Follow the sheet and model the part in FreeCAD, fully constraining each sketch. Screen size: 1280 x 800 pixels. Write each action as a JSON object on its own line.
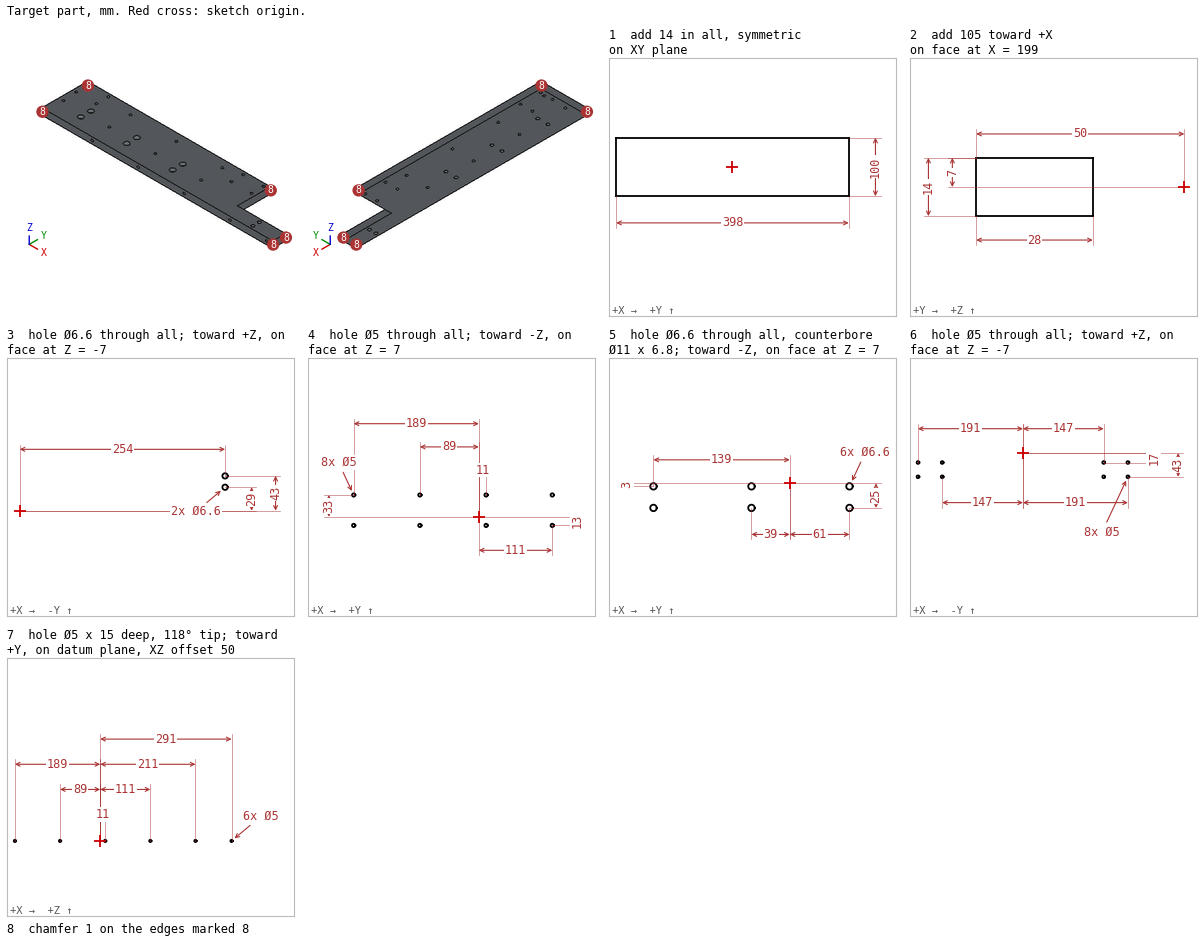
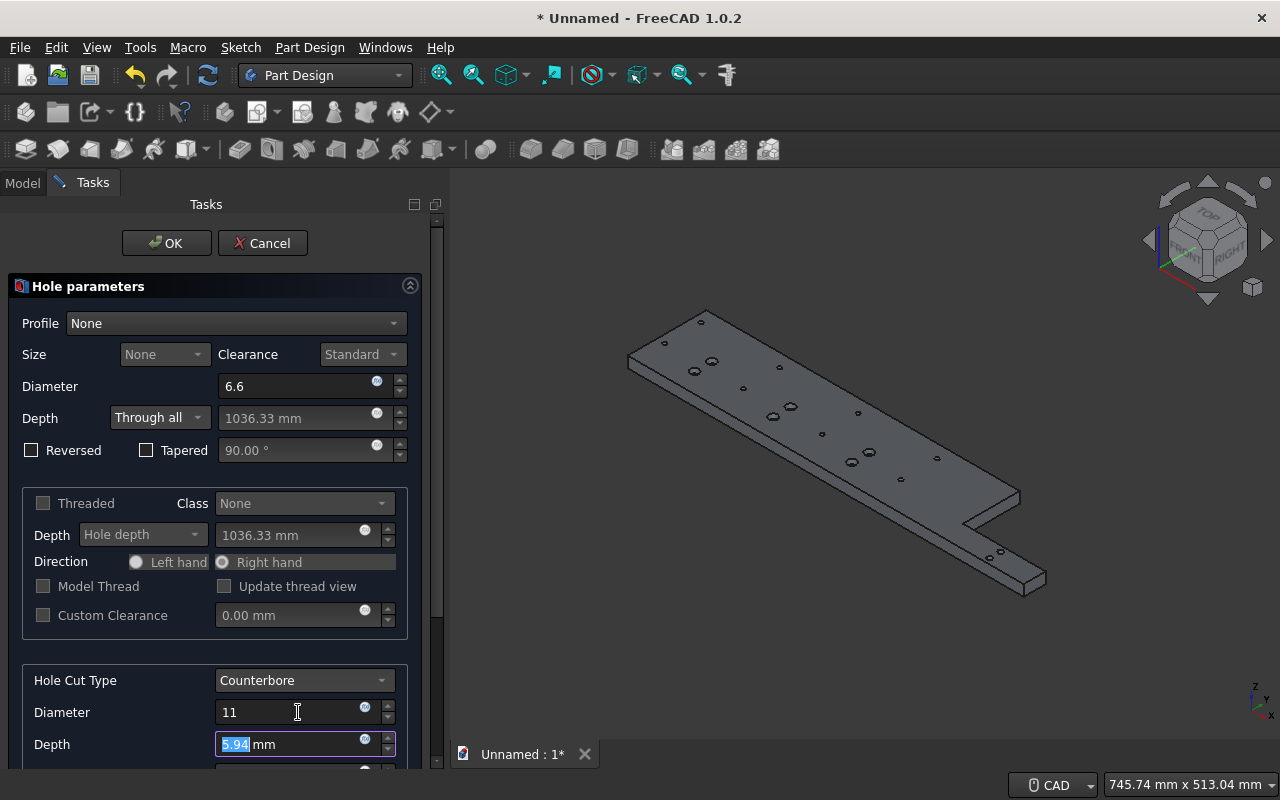
{"action": "type", "text": "6.8"}
{"action": "key", "text": "Tab"}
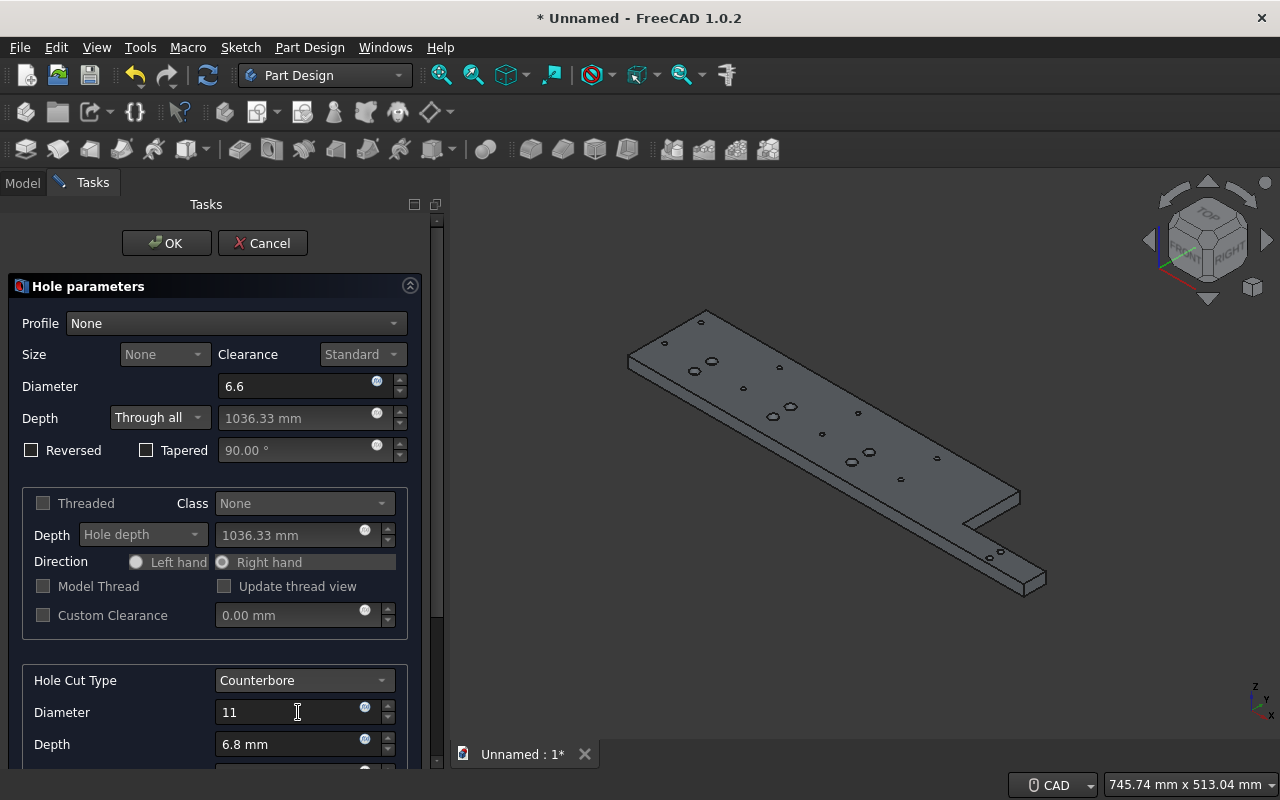
{"action": "left_click", "coordinate": [167, 243]}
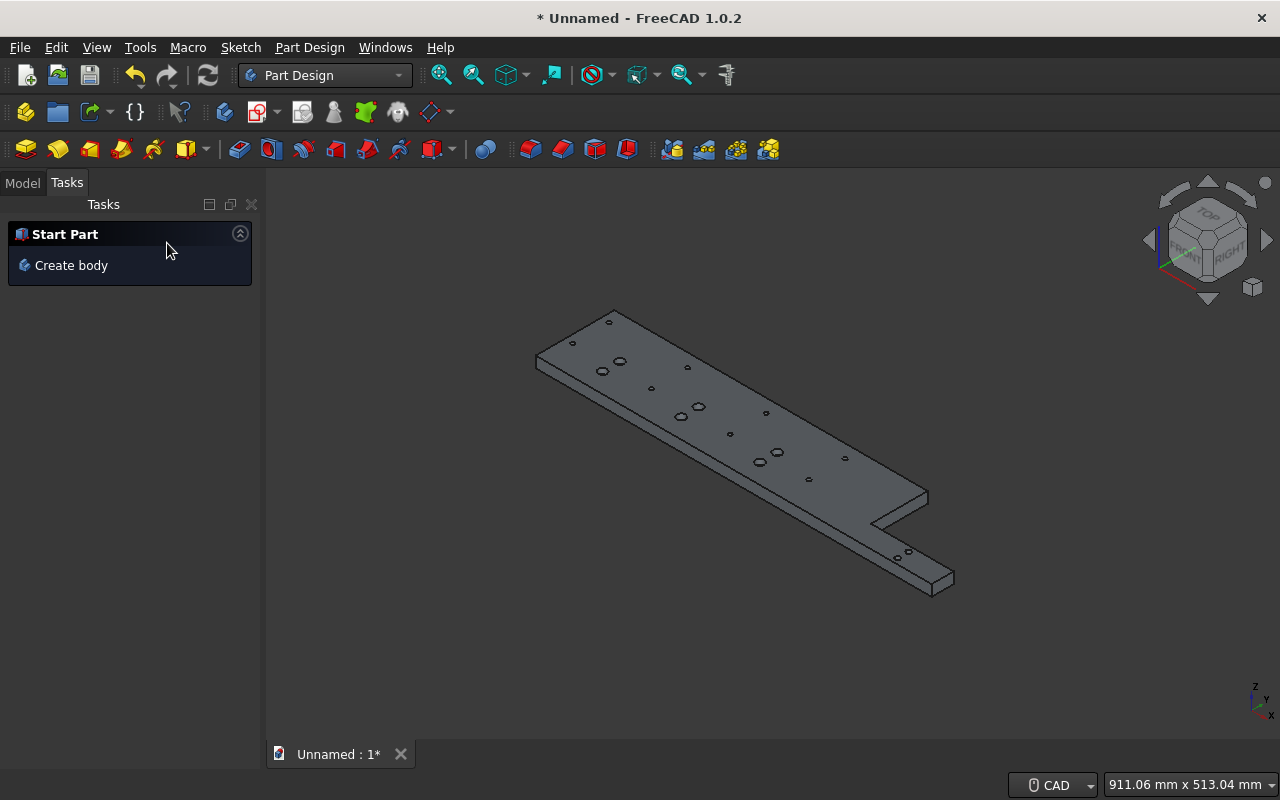
{"action": "key", "text": "5"}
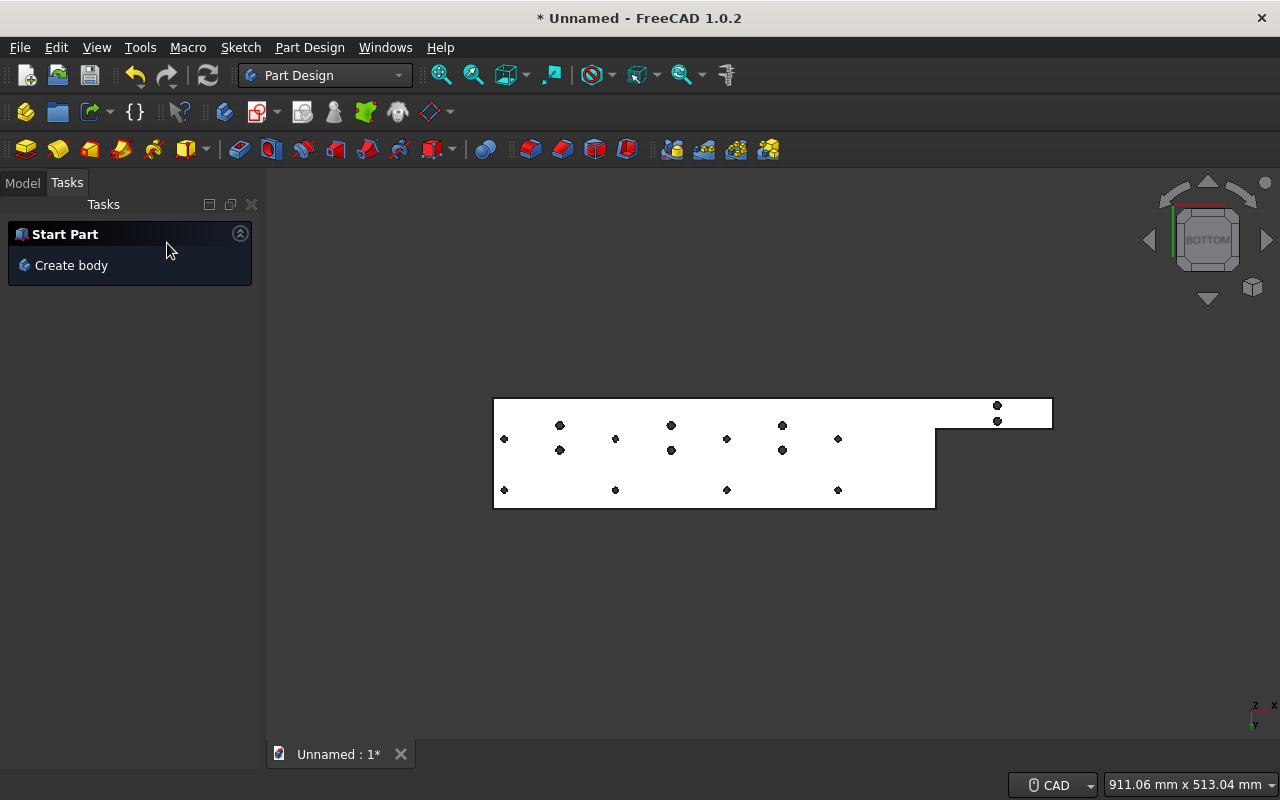
{"action": "left_click", "coordinate": [533, 468]}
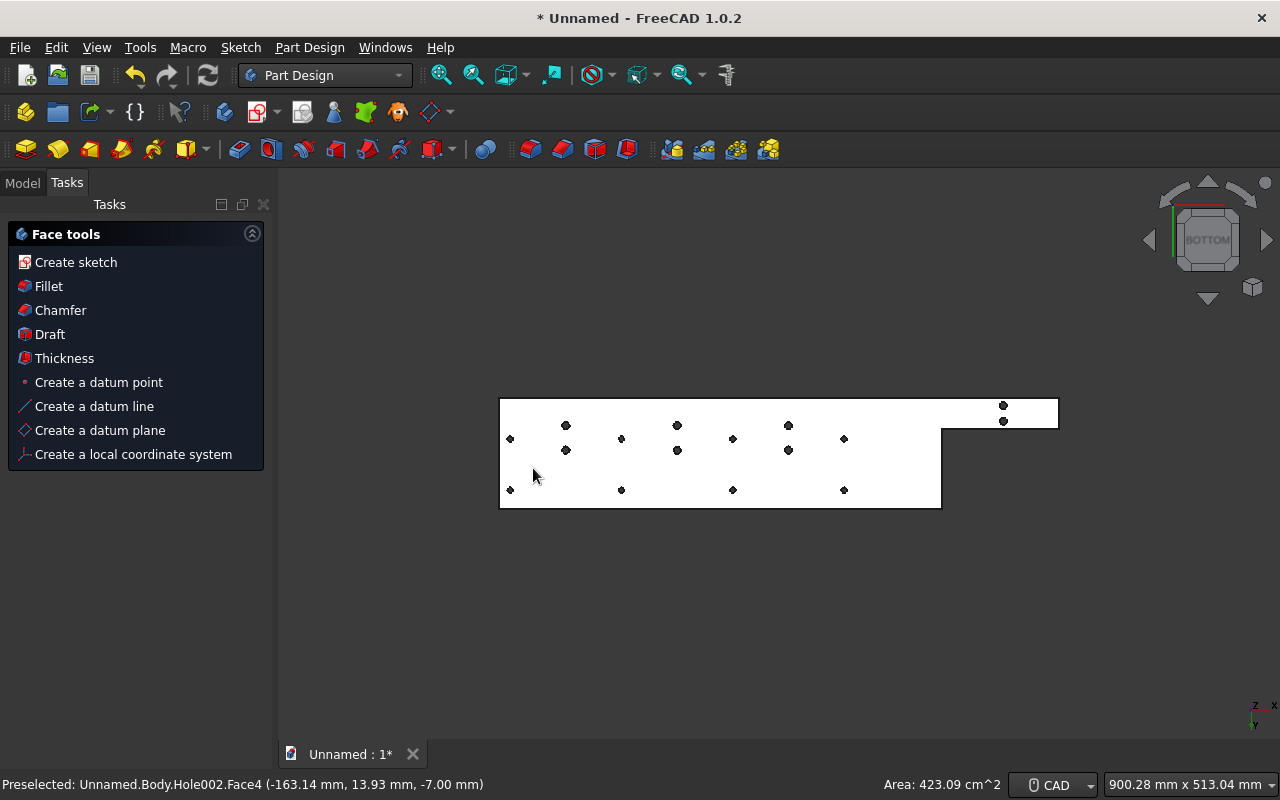
{"action": "left_click", "coordinate": [258, 112]}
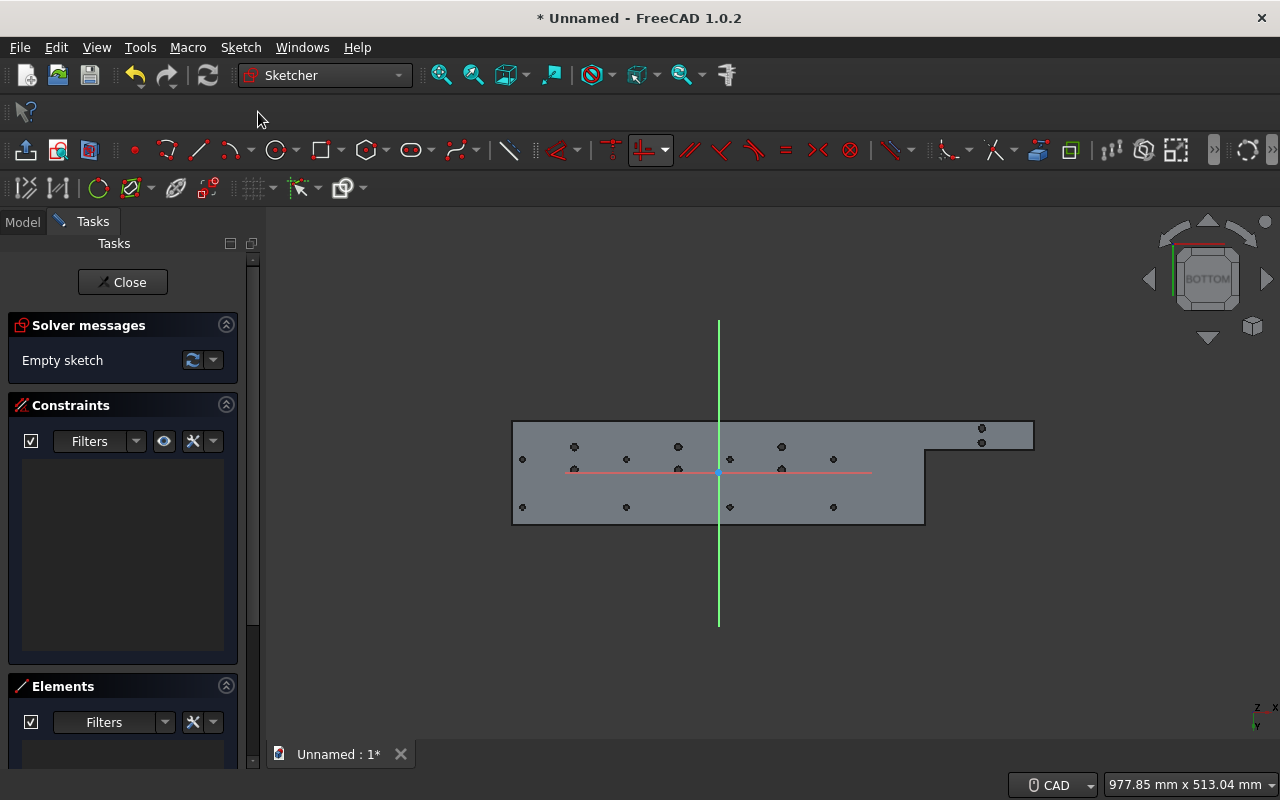
{"action": "scroll", "coordinate": [747, 545], "scroll_direction": "up", "scroll_amount": 2}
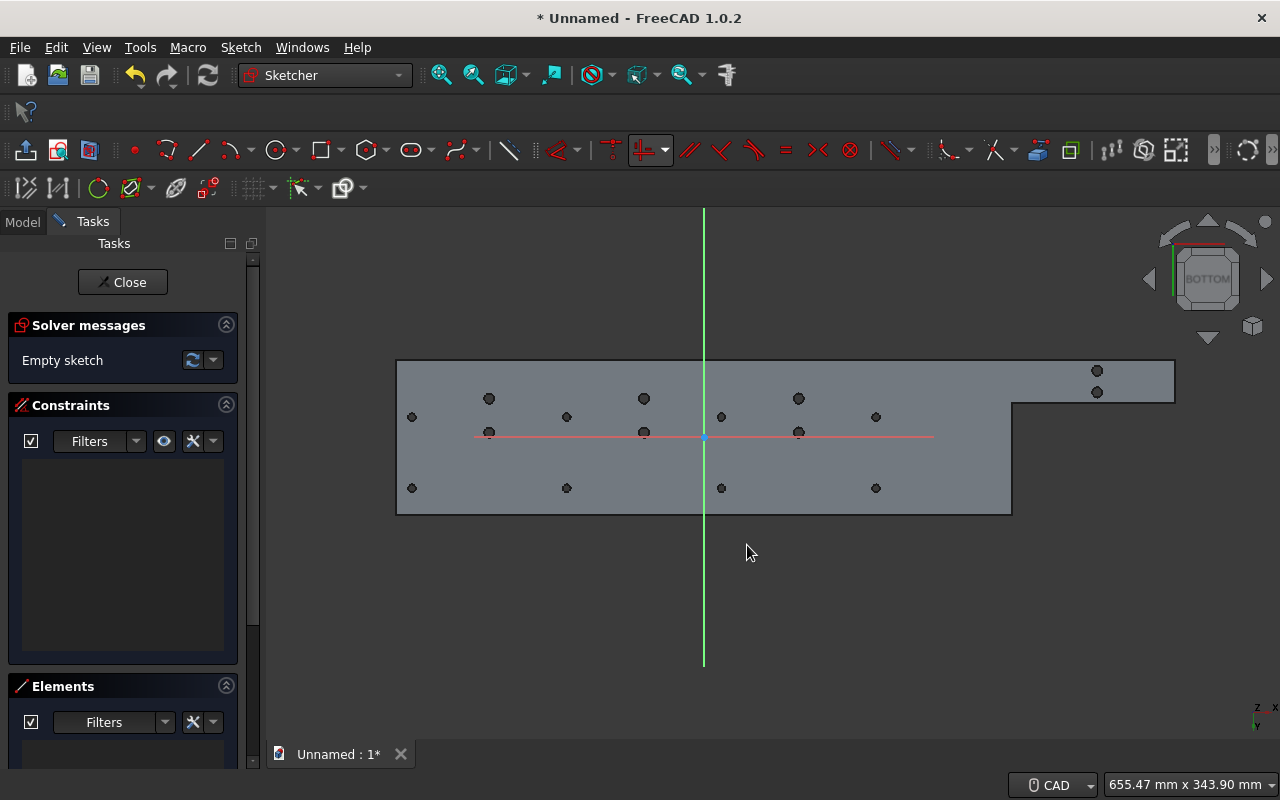
{"action": "key", "text": "g c"}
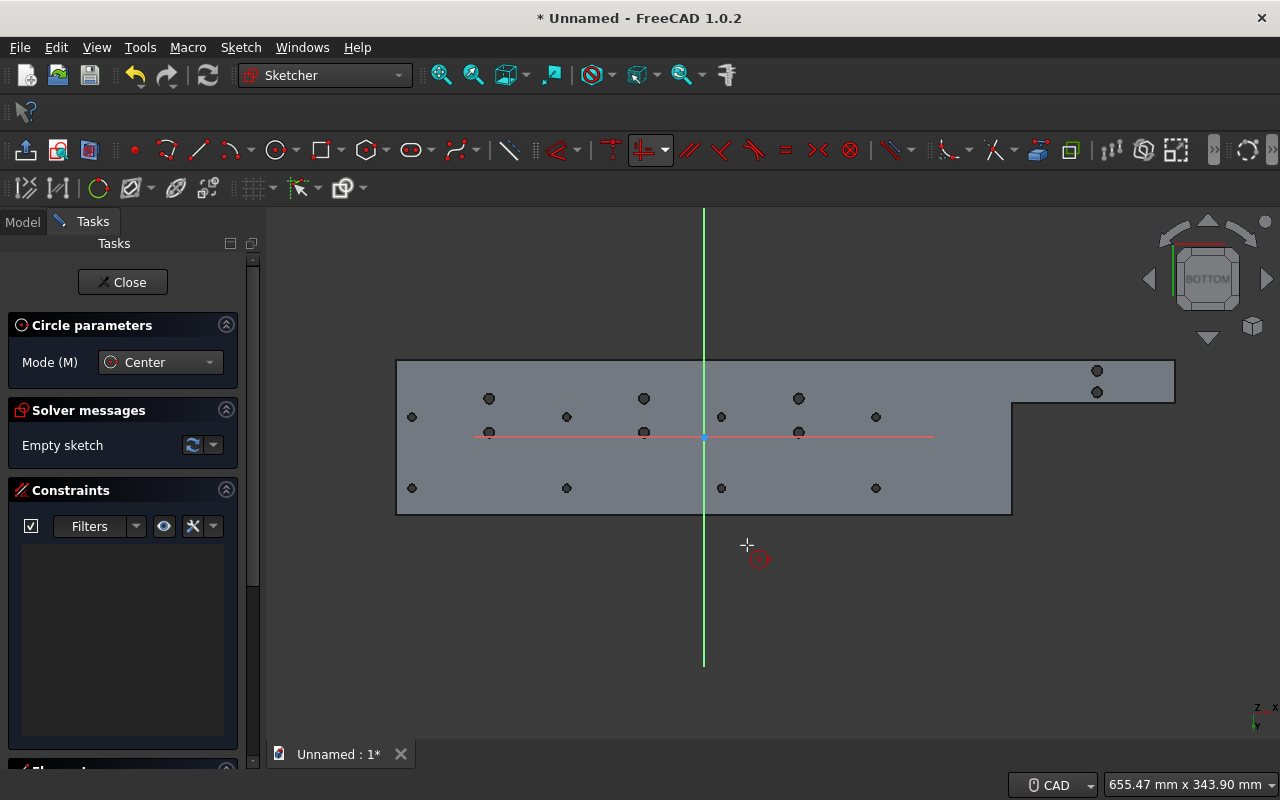
{"action": "scroll", "coordinate": [1000, 504], "scroll_direction": "up", "scroll_amount": 9}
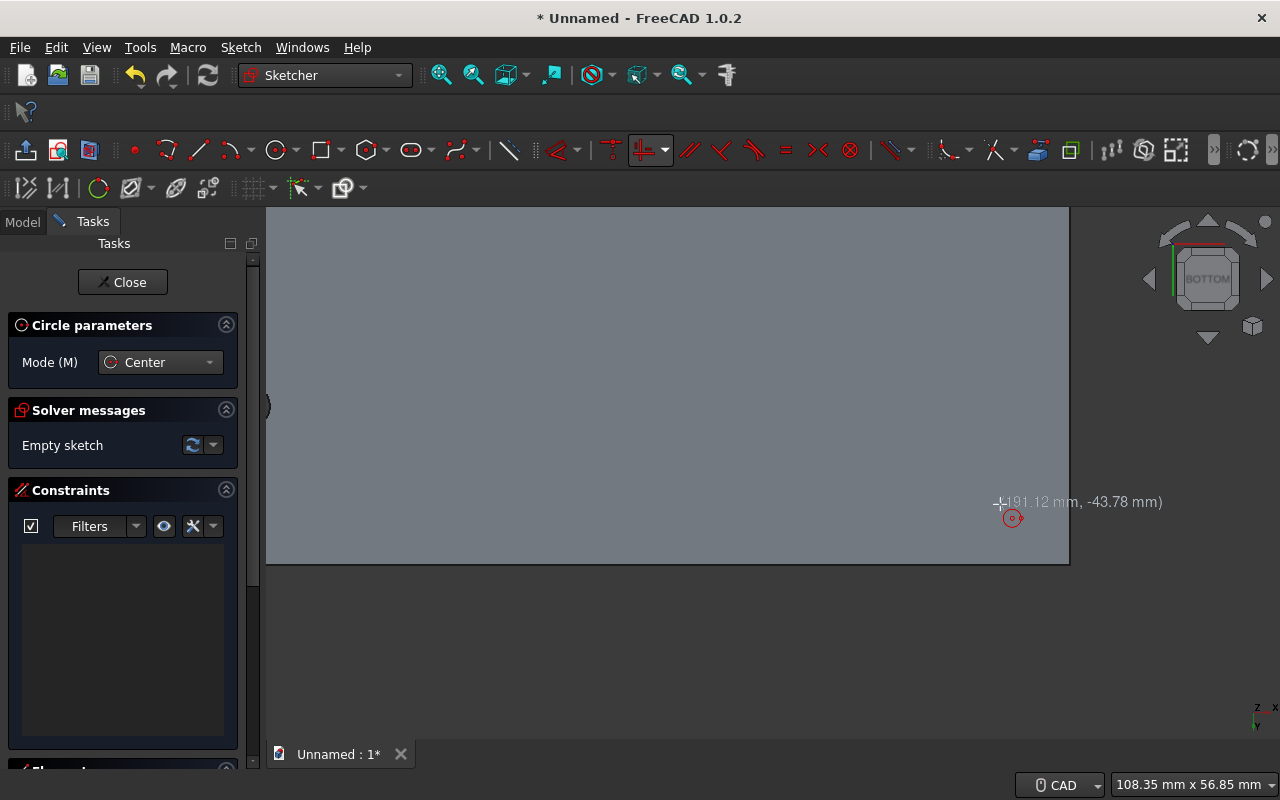
{"action": "scroll", "coordinate": [1001, 505], "scroll_direction": "down", "scroll_amount": 9}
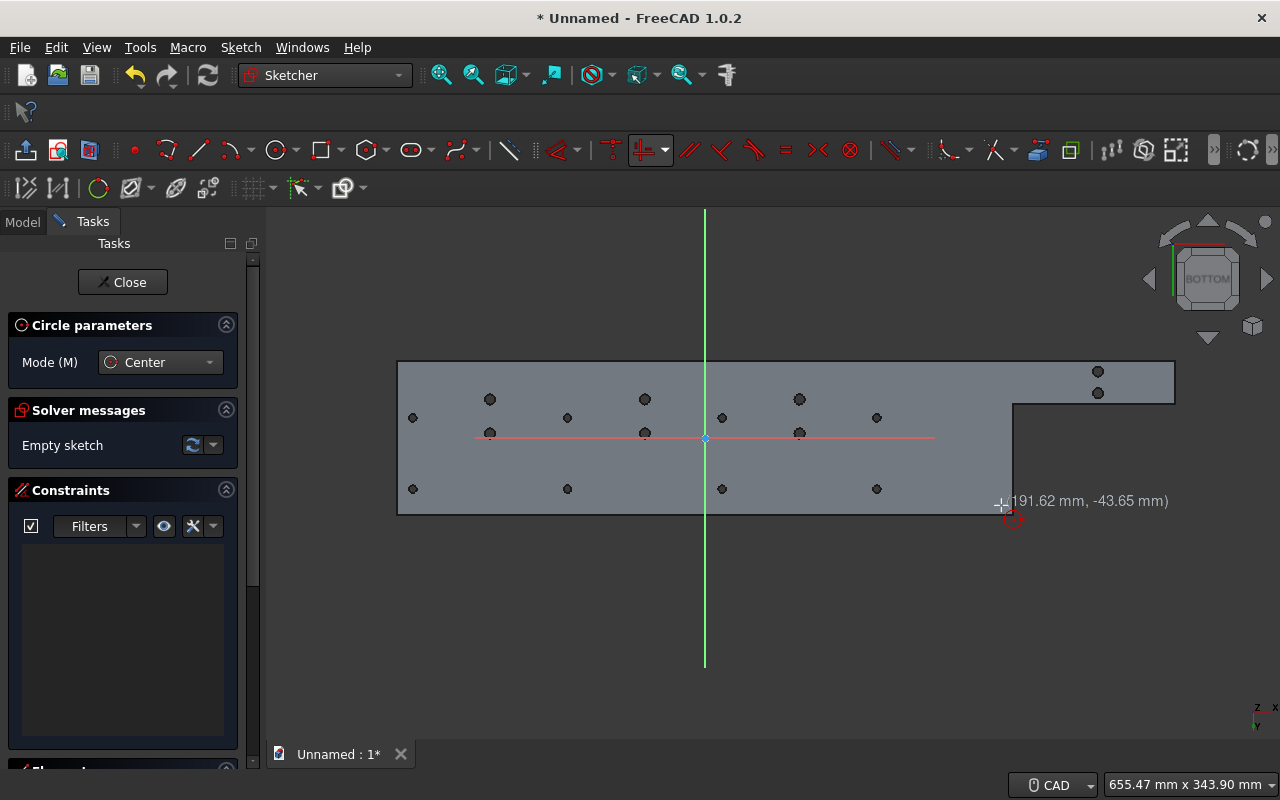
{"action": "left_click", "coordinate": [1001, 505]}